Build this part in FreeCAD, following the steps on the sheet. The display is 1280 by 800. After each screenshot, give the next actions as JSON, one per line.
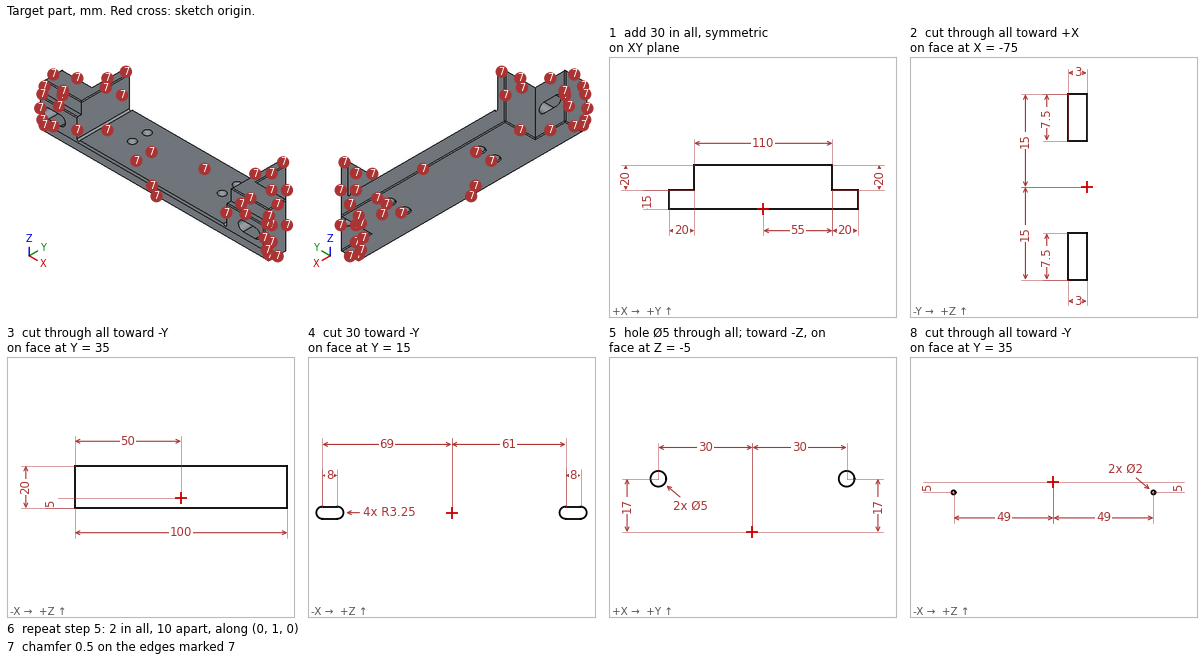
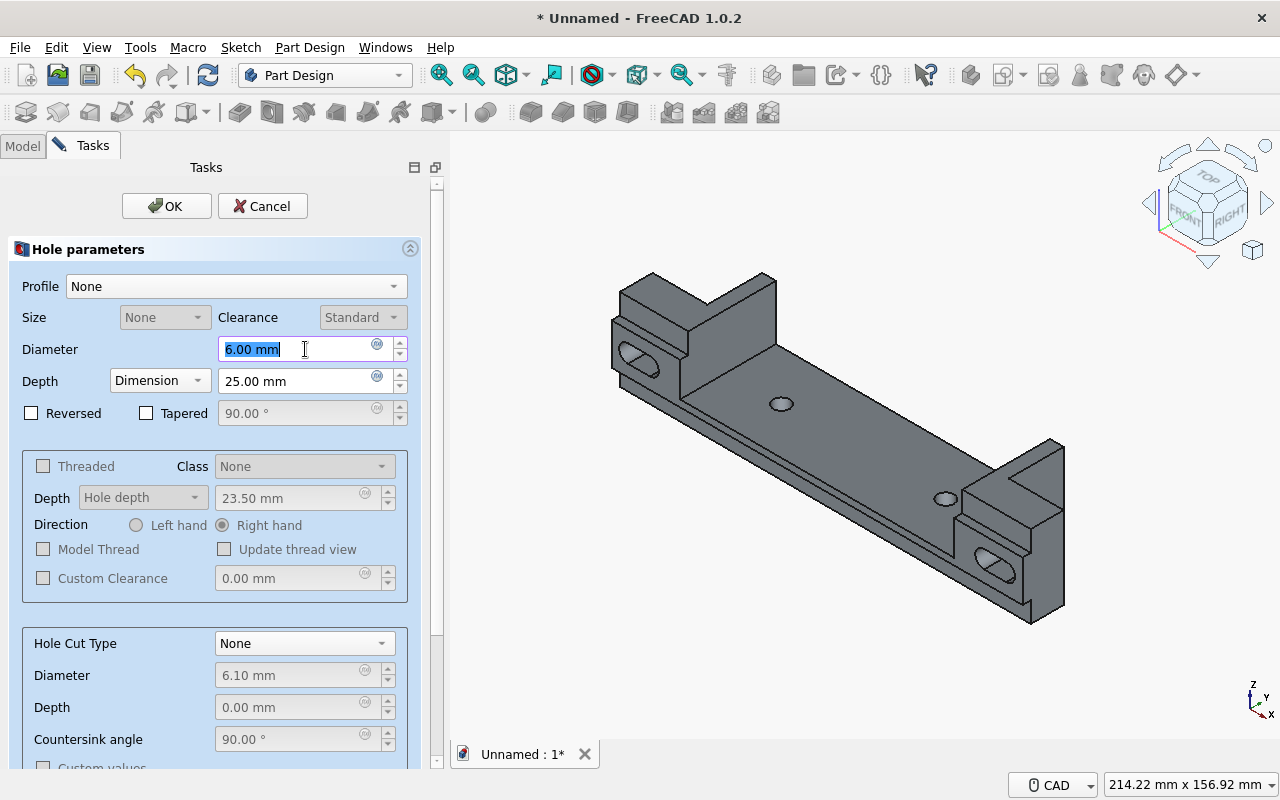
{"action": "type", "text": "5"}
{"action": "key", "text": "Tab"}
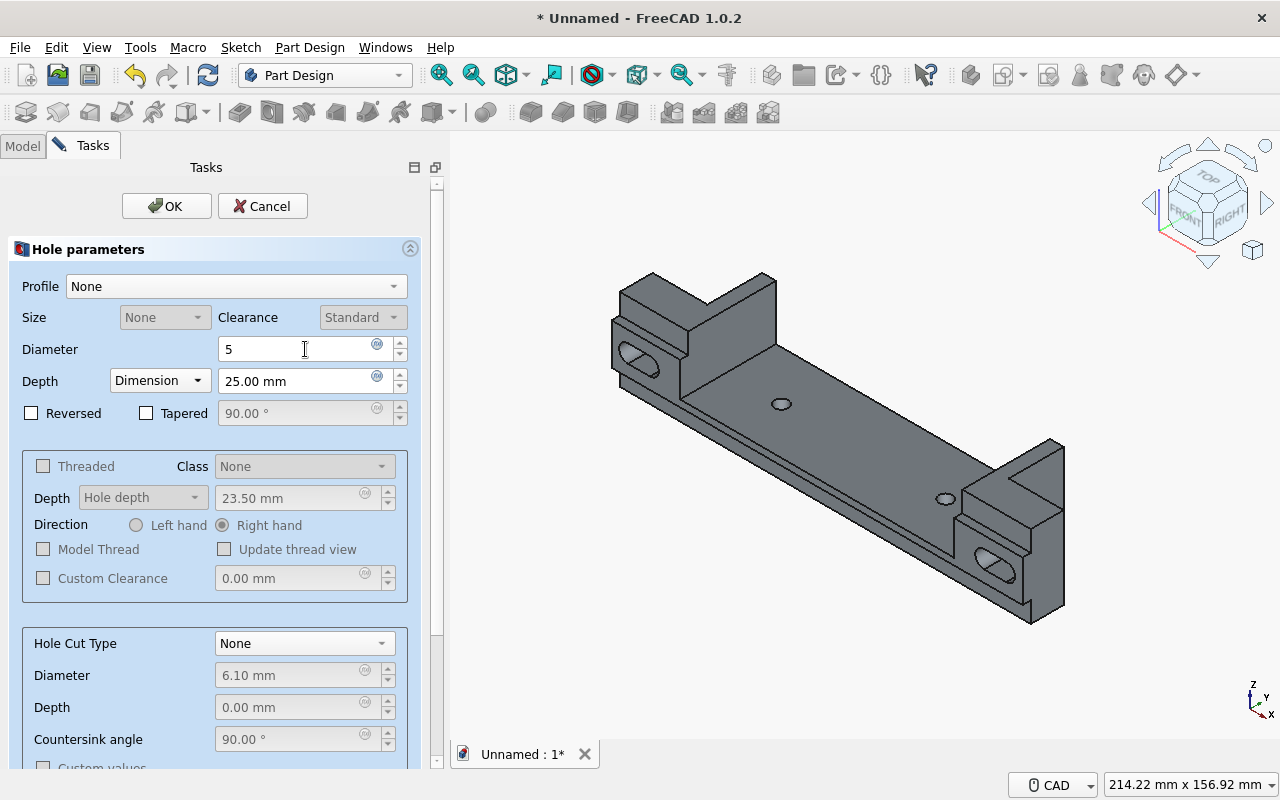
{"action": "left_click", "coordinate": [161, 380]}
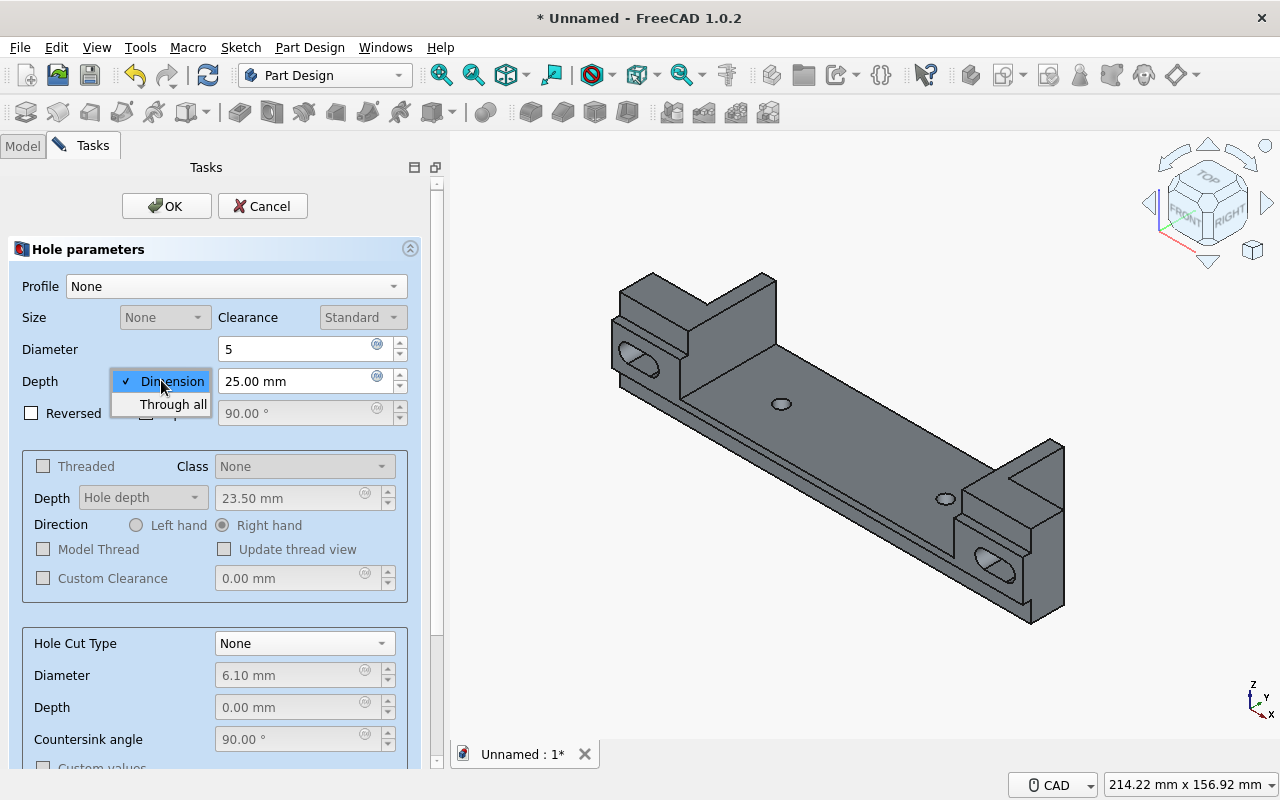
{"action": "left_click", "coordinate": [160, 404]}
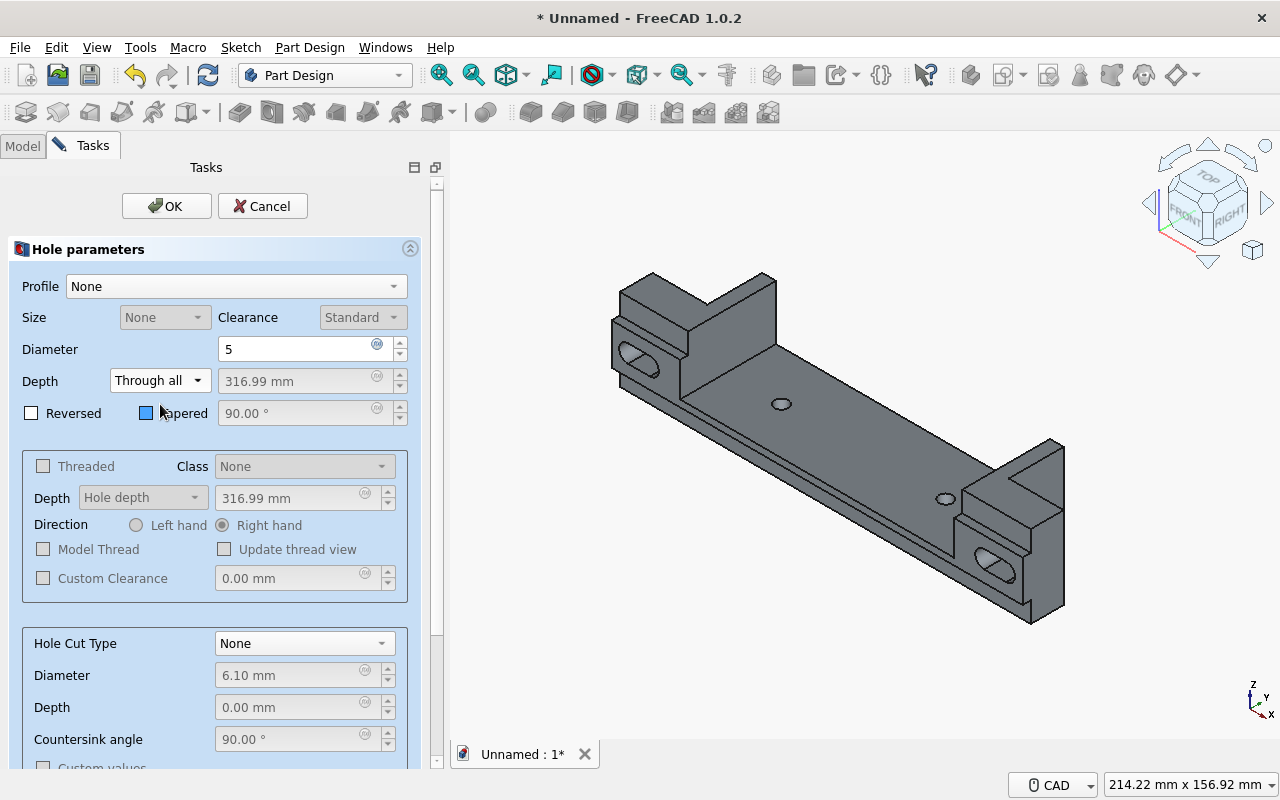
{"action": "left_click", "coordinate": [167, 206]}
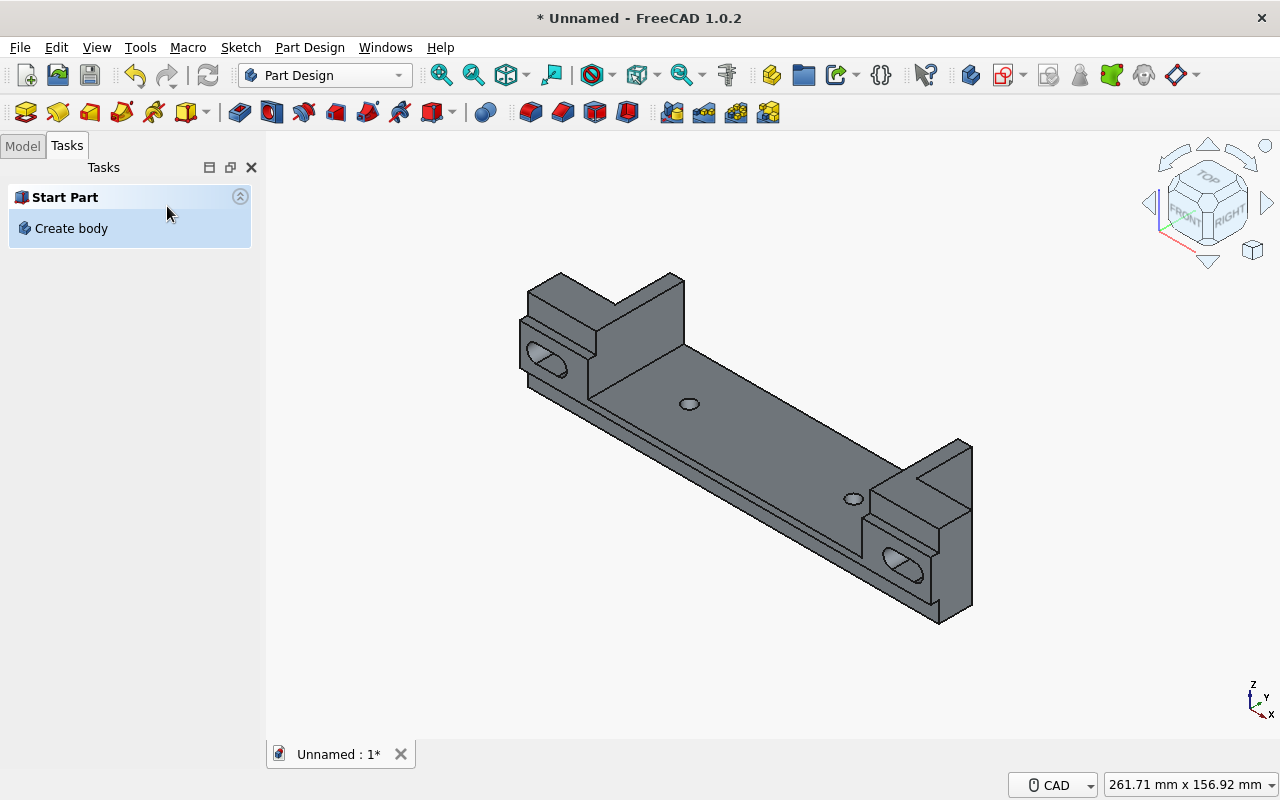
{"action": "left_click", "coordinate": [23, 145]}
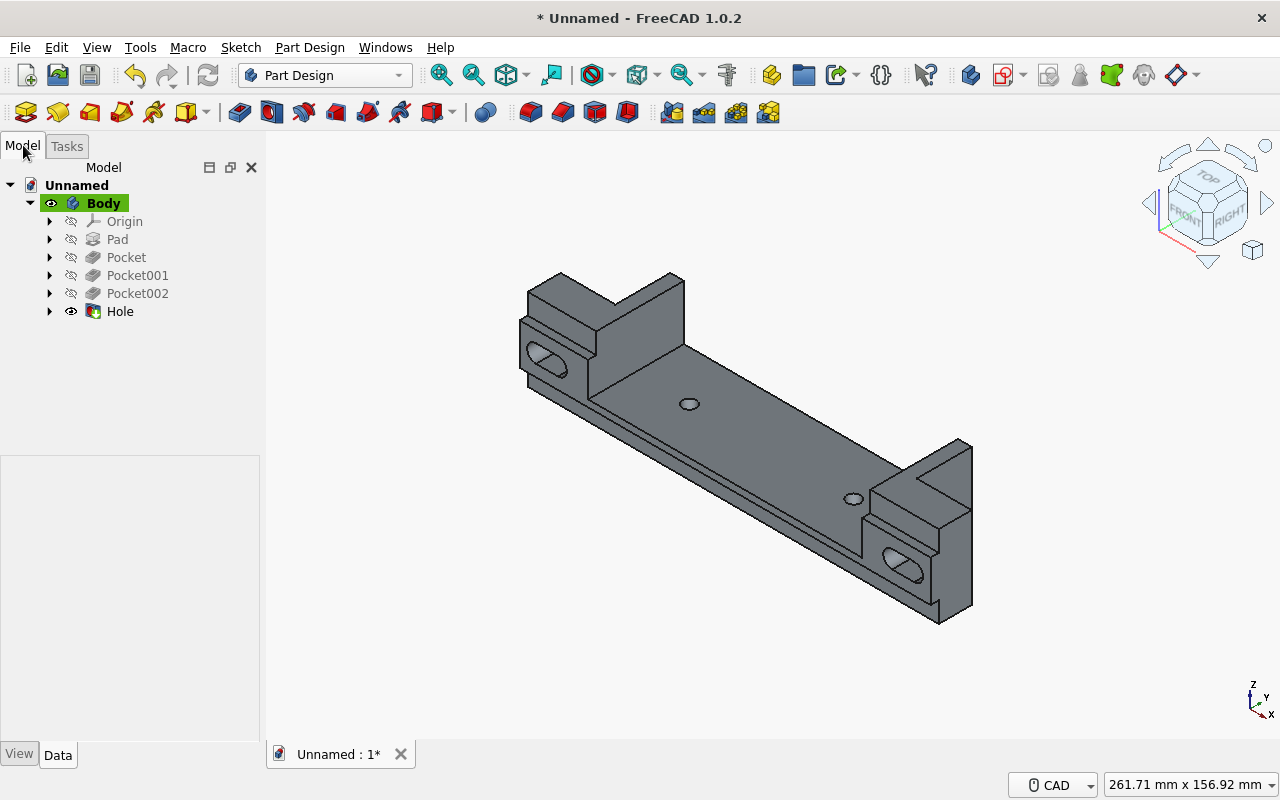
{"action": "left_click", "coordinate": [116, 311]}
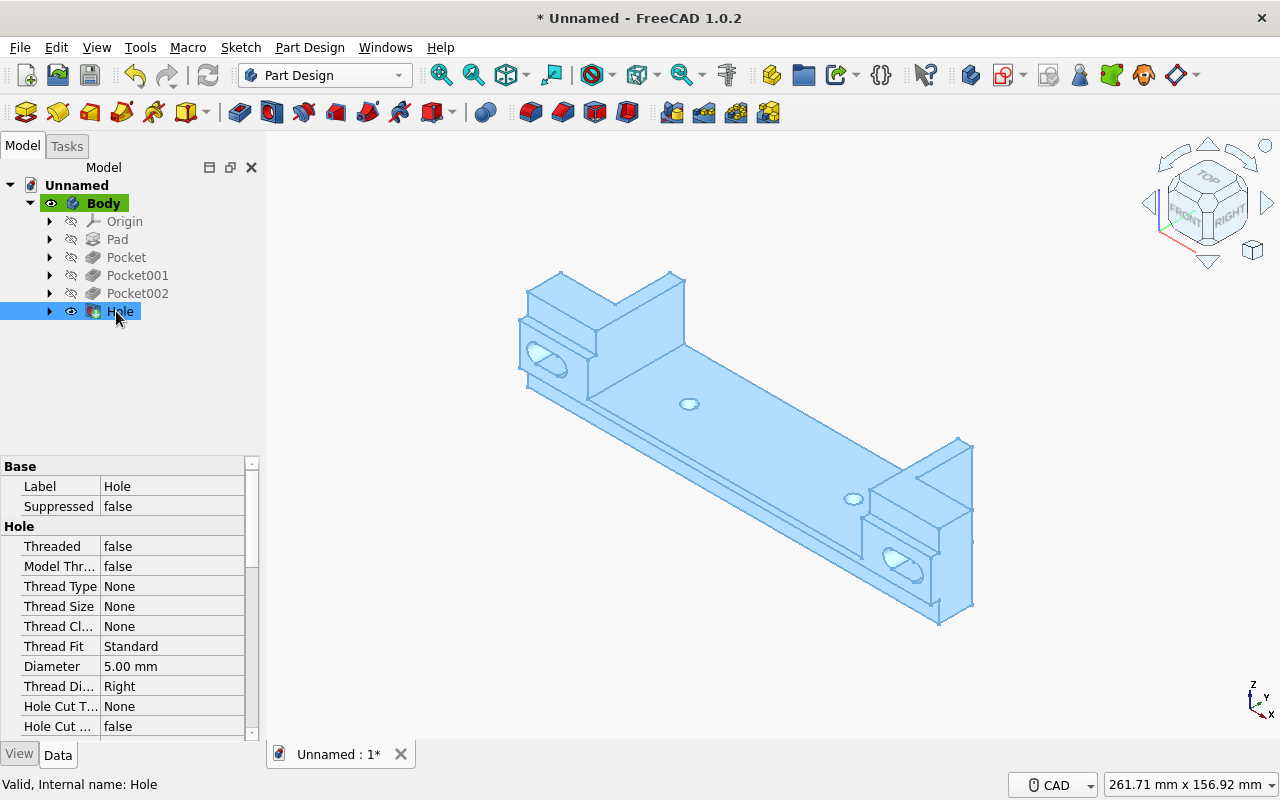
{"action": "left_click", "coordinate": [704, 112]}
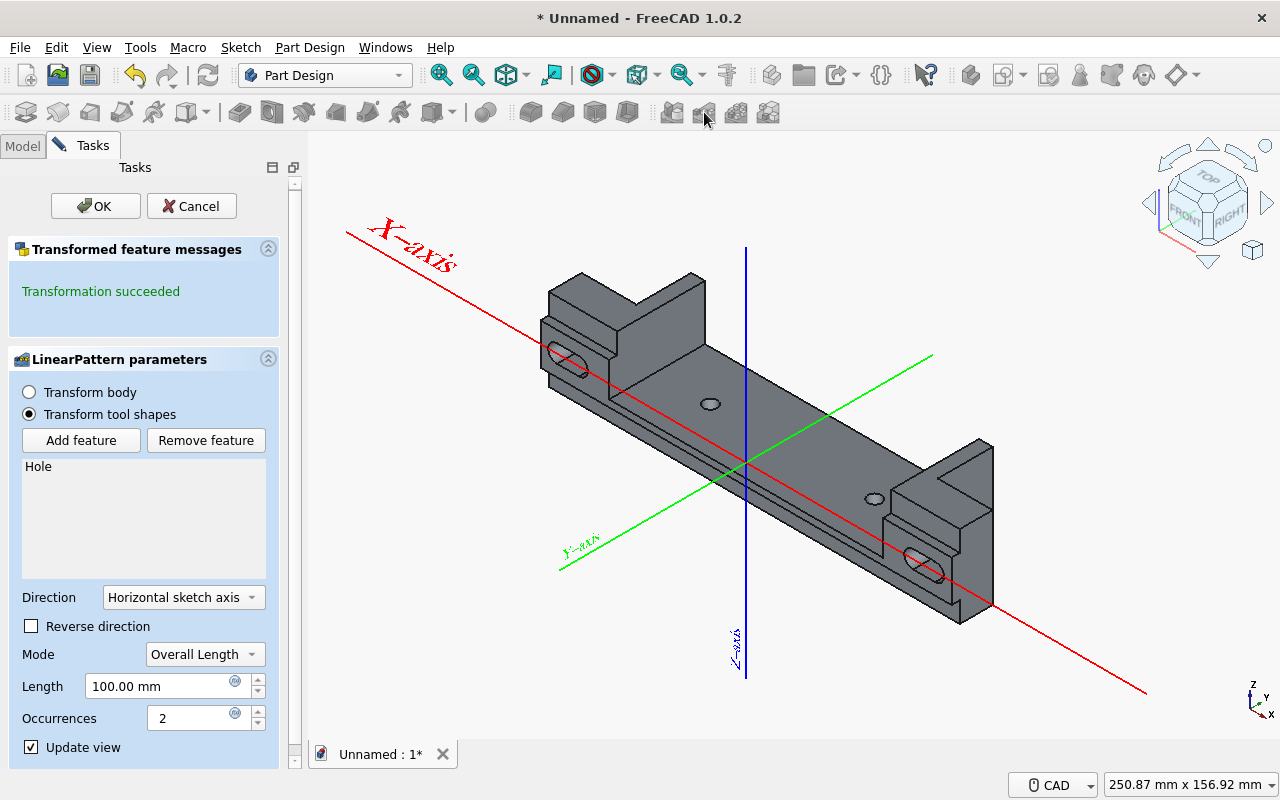
{"action": "left_click", "coordinate": [184, 598]}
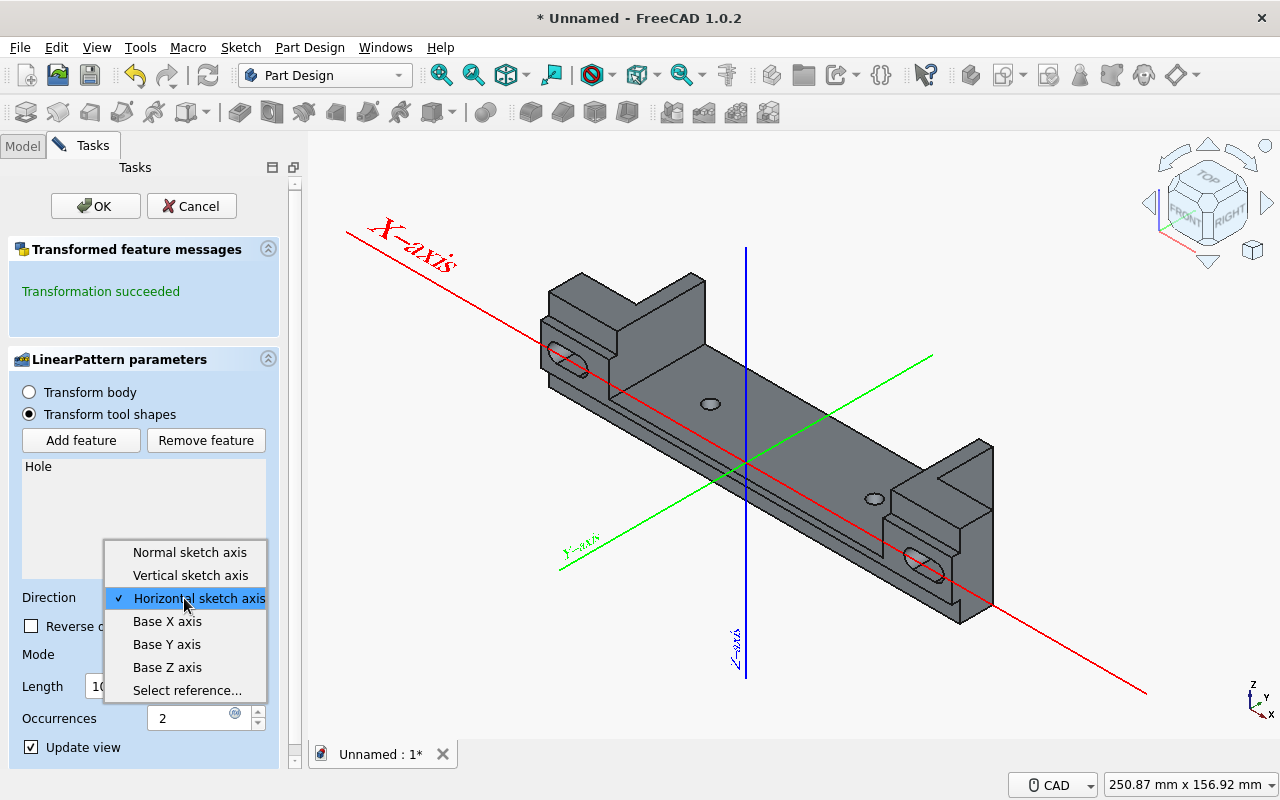
{"action": "left_click", "coordinate": [184, 644]}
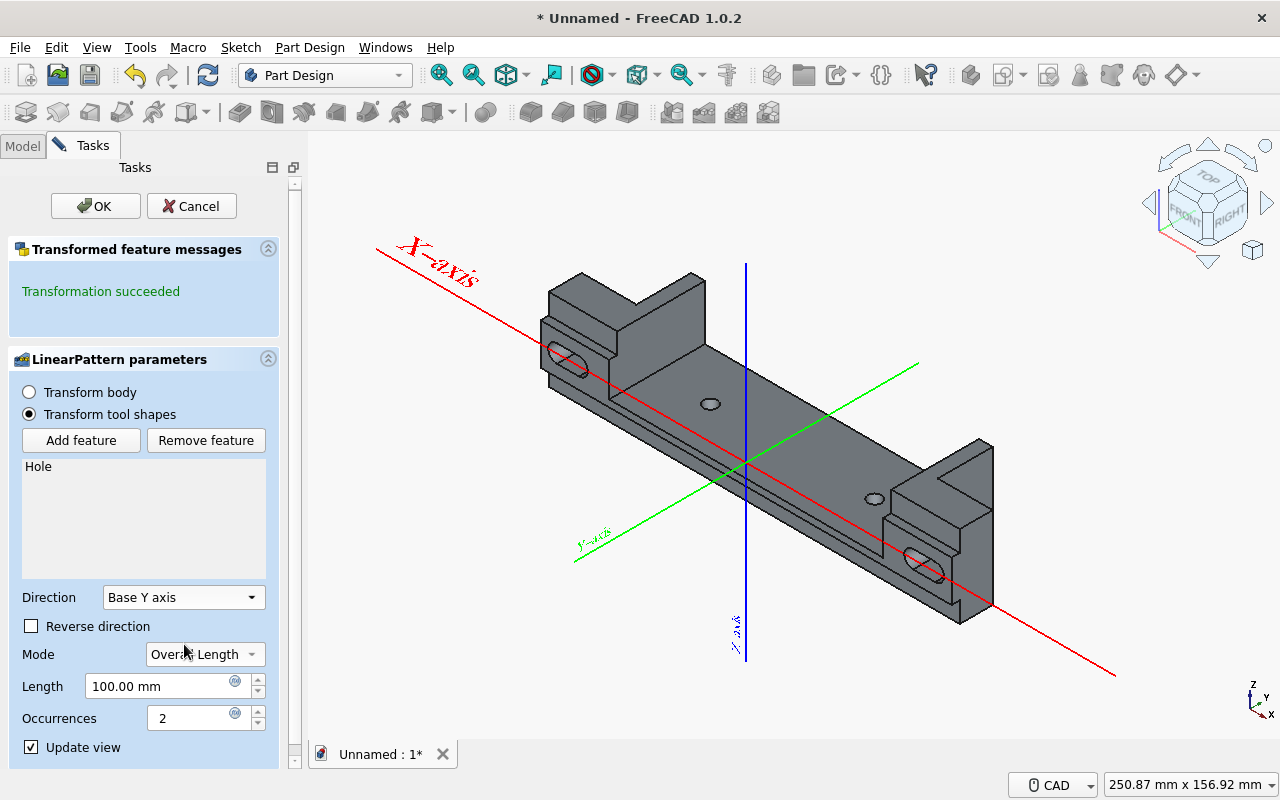
{"action": "left_click", "coordinate": [206, 654]}